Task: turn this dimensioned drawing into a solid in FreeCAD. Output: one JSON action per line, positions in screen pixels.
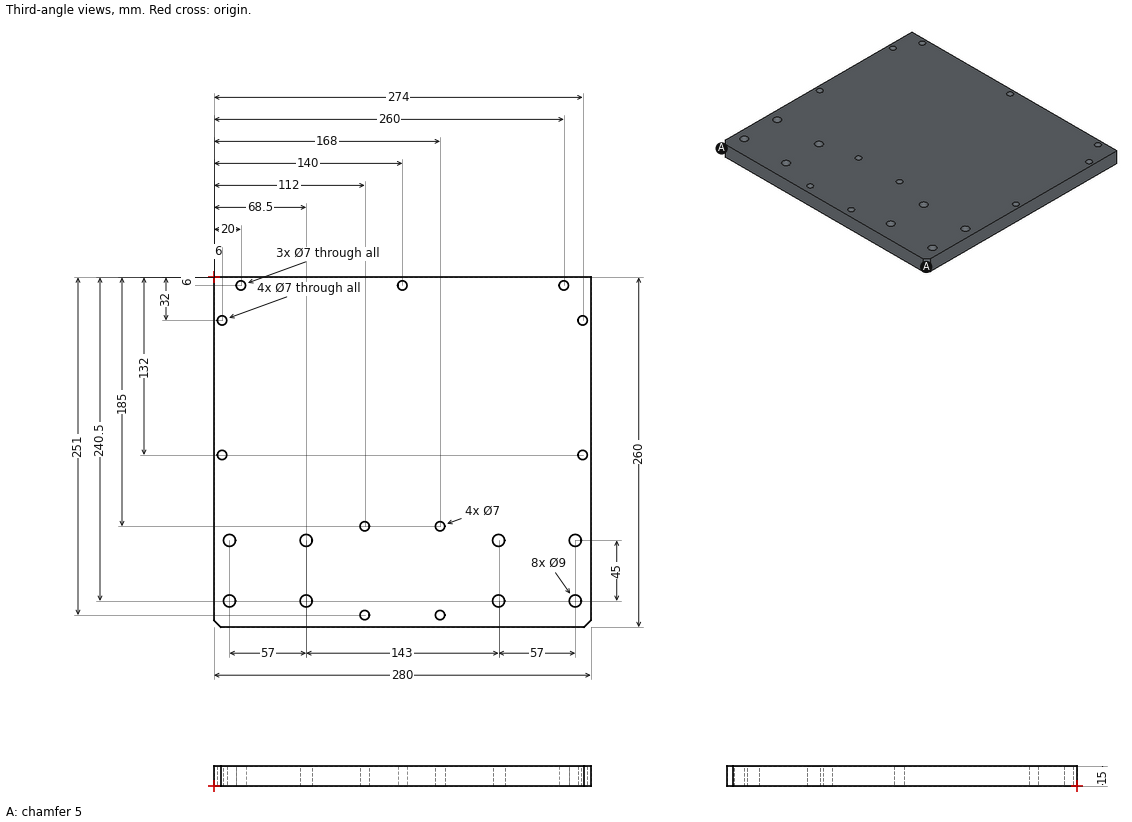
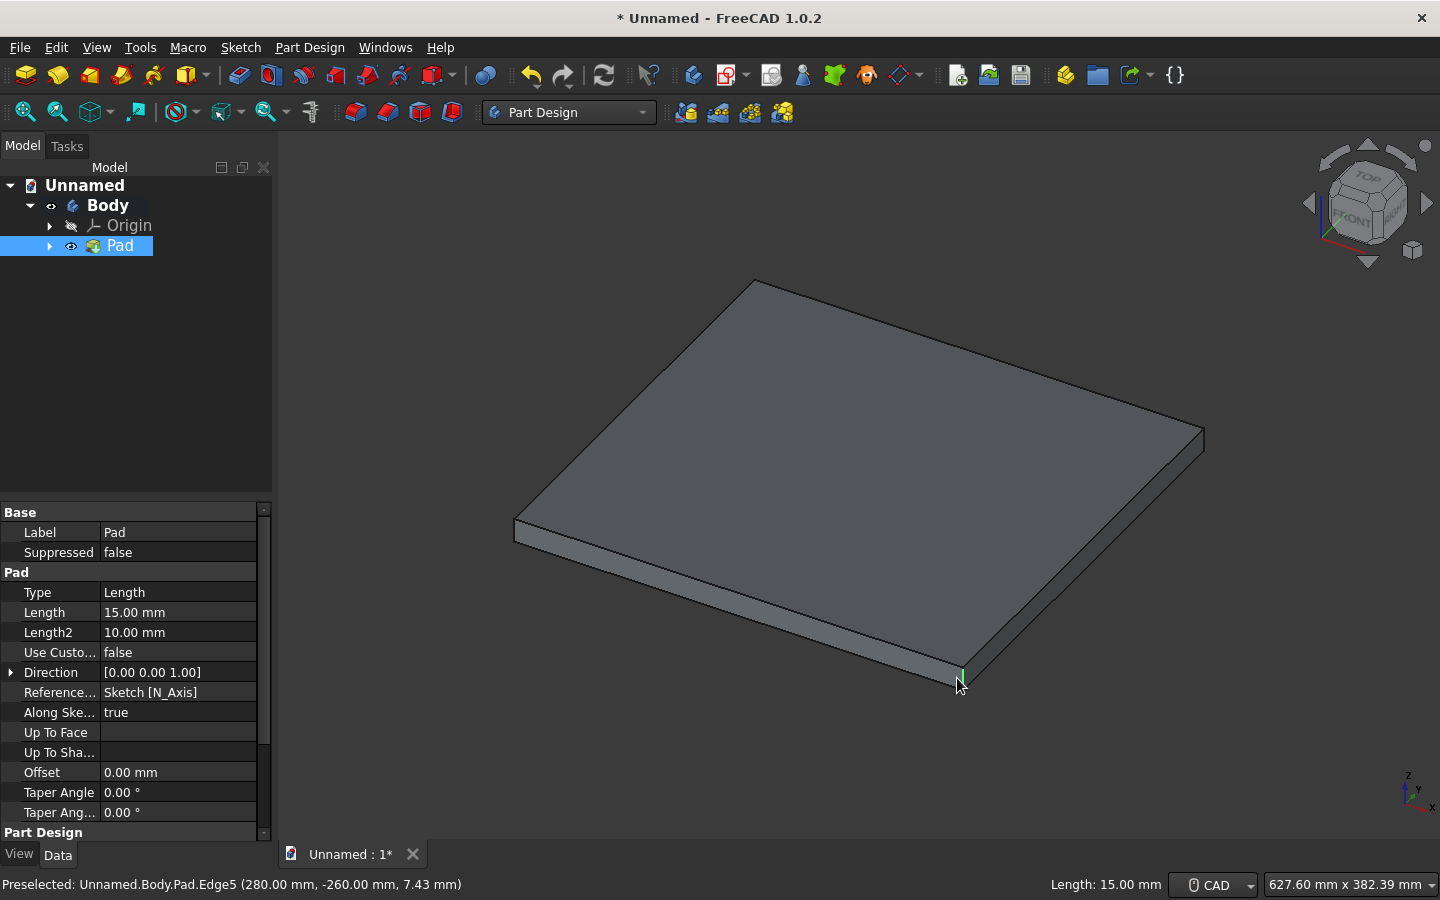
{"action": "key", "text": "0"}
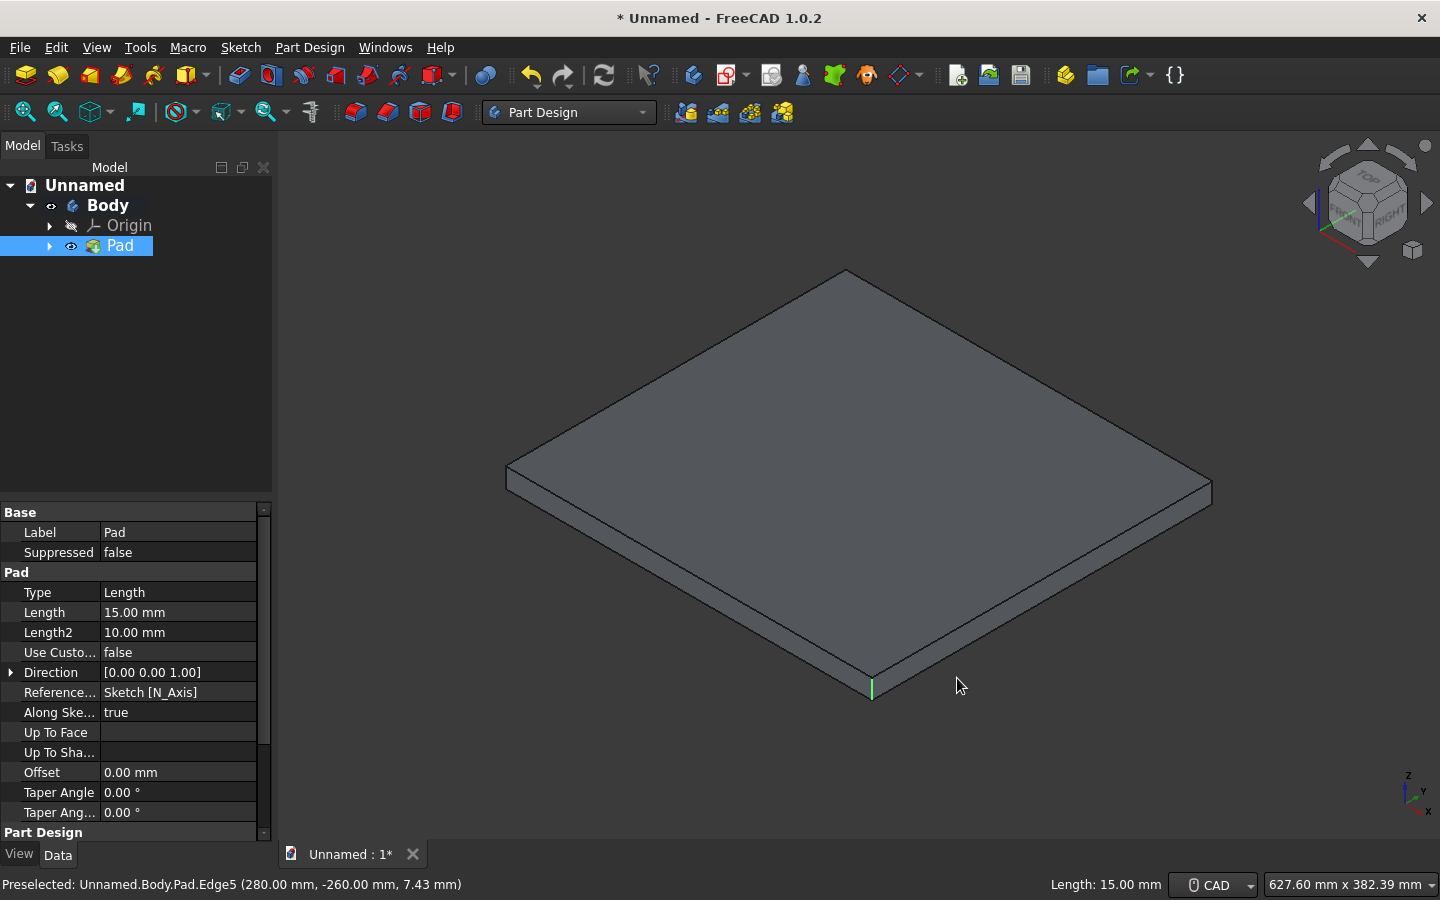
{"action": "key", "text": "2"}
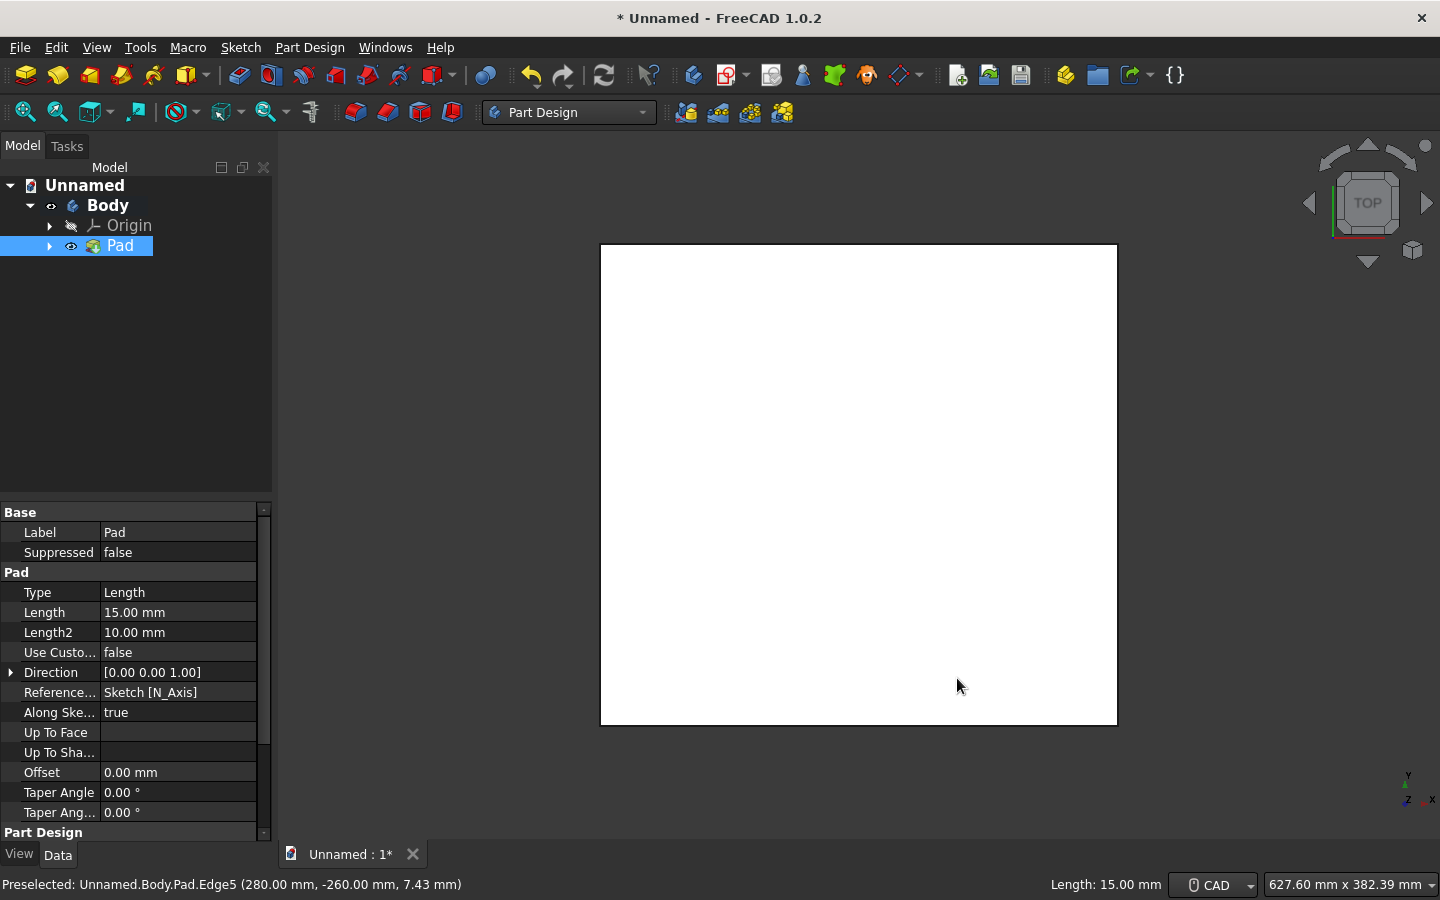
{"action": "key", "text": "1"}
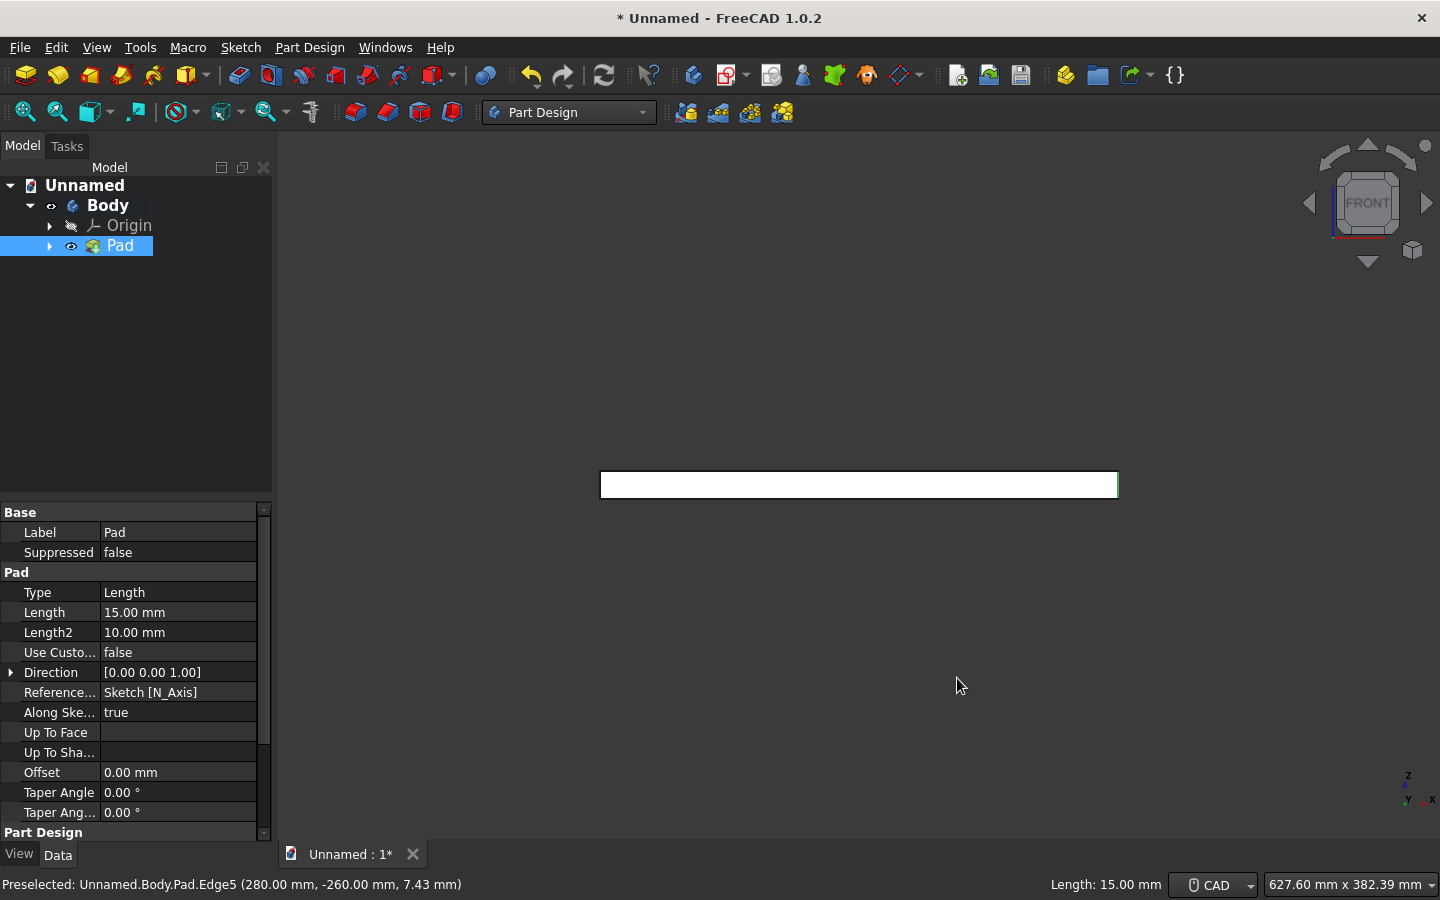
{"action": "left_click", "coordinate": [26, 112]}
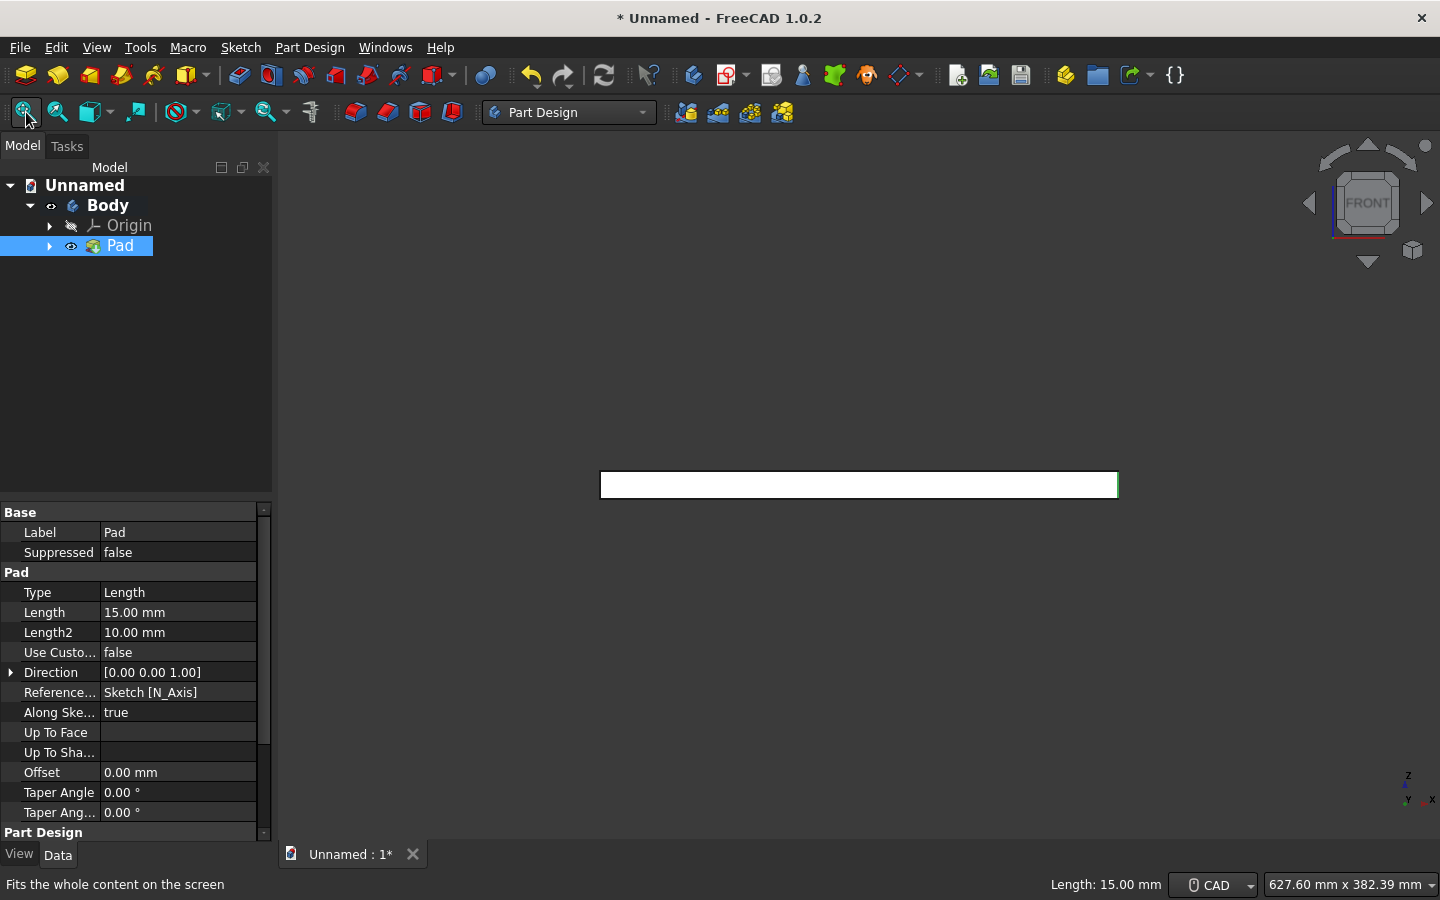
{"action": "left_click", "coordinate": [600, 484], "text": "ctrl"}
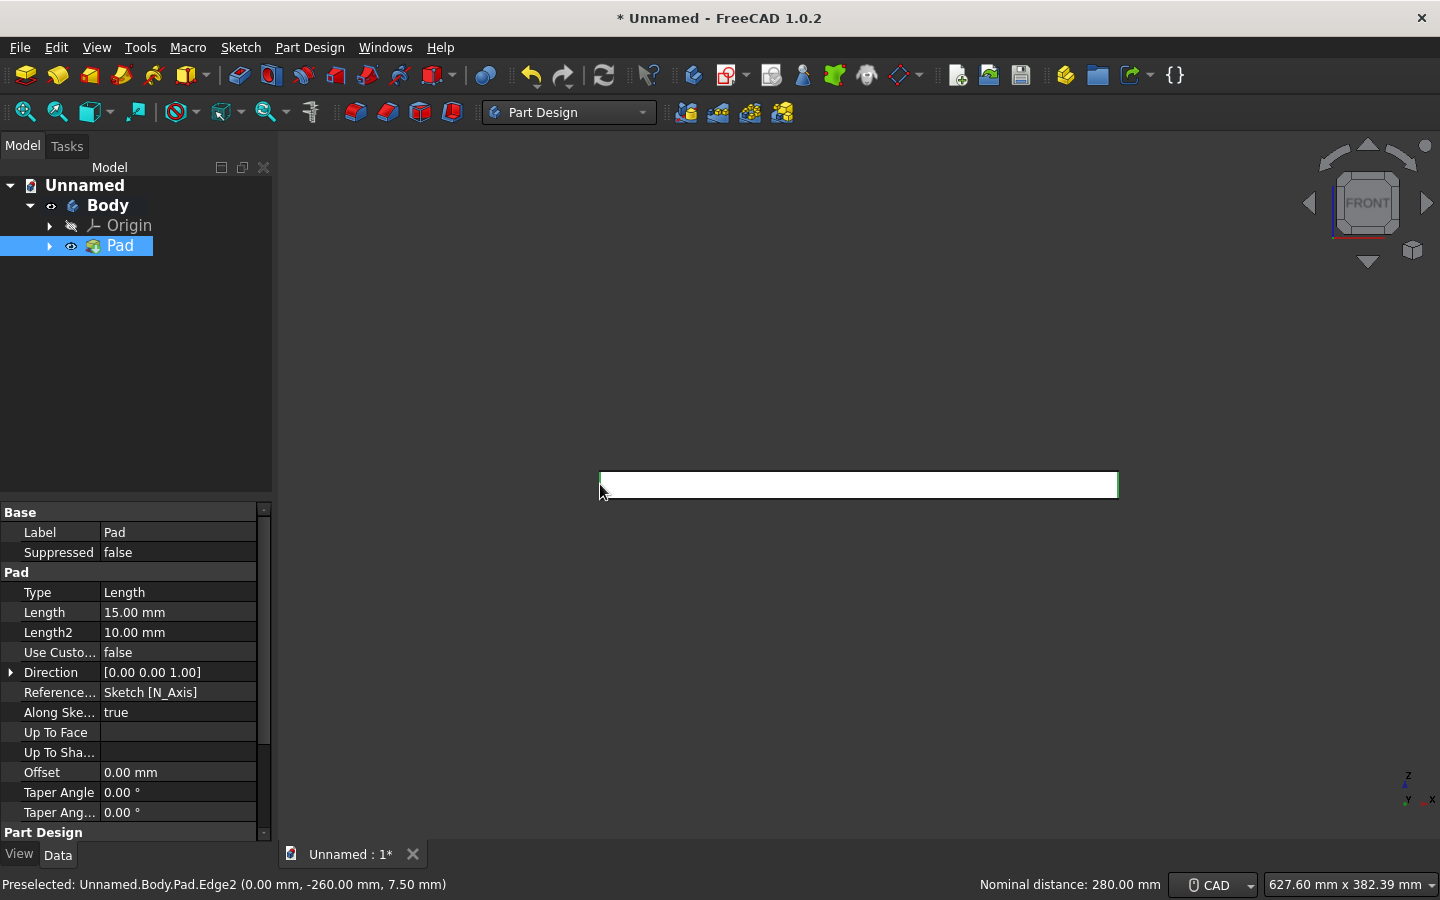
{"action": "left_click", "coordinate": [388, 112]}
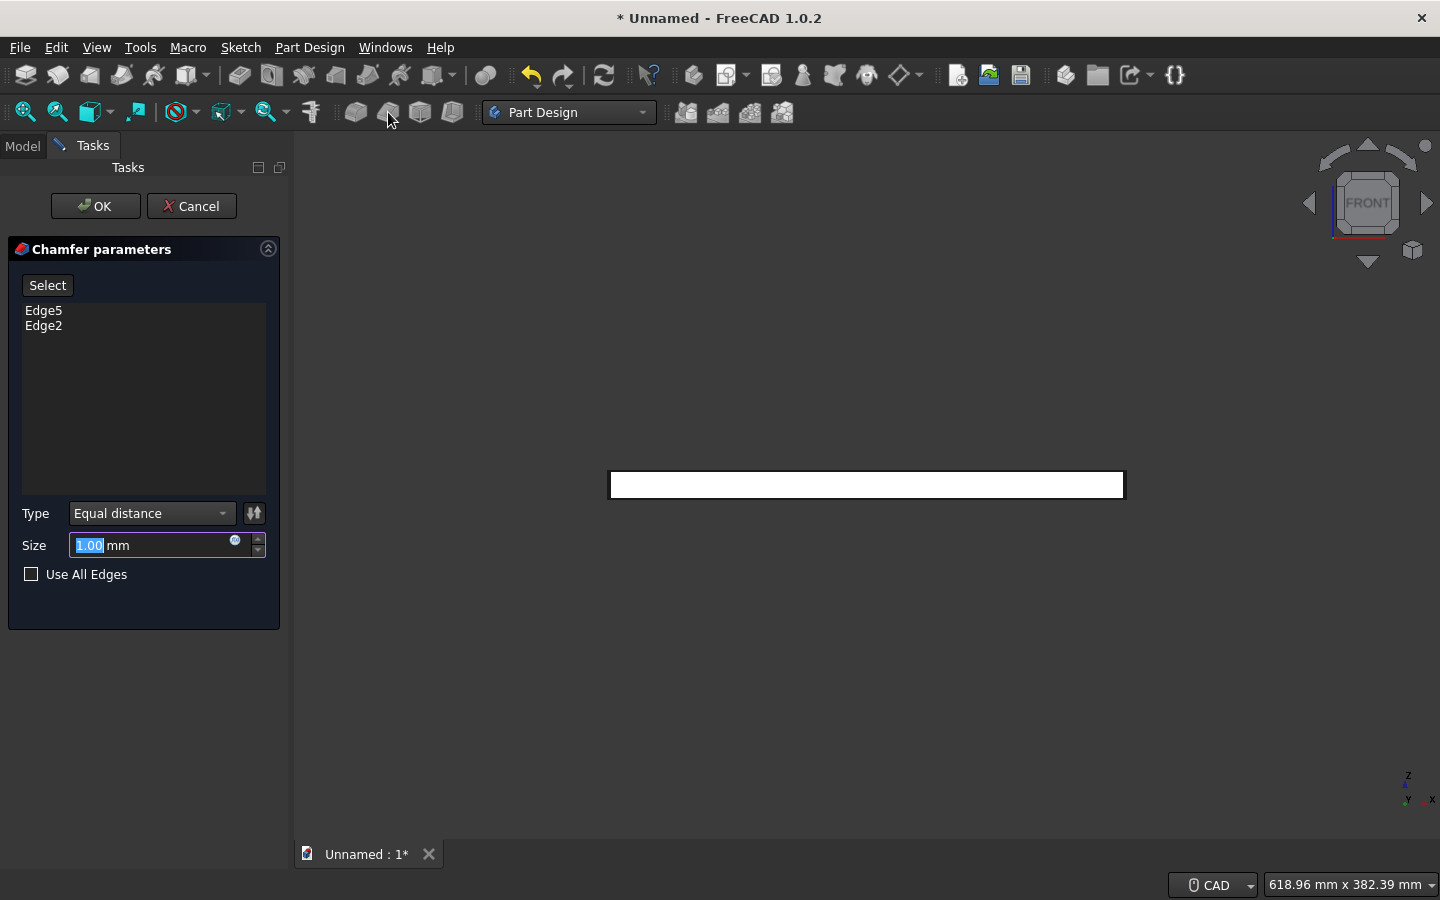
{"action": "type", "text": "5"}
{"action": "key", "text": "Tab"}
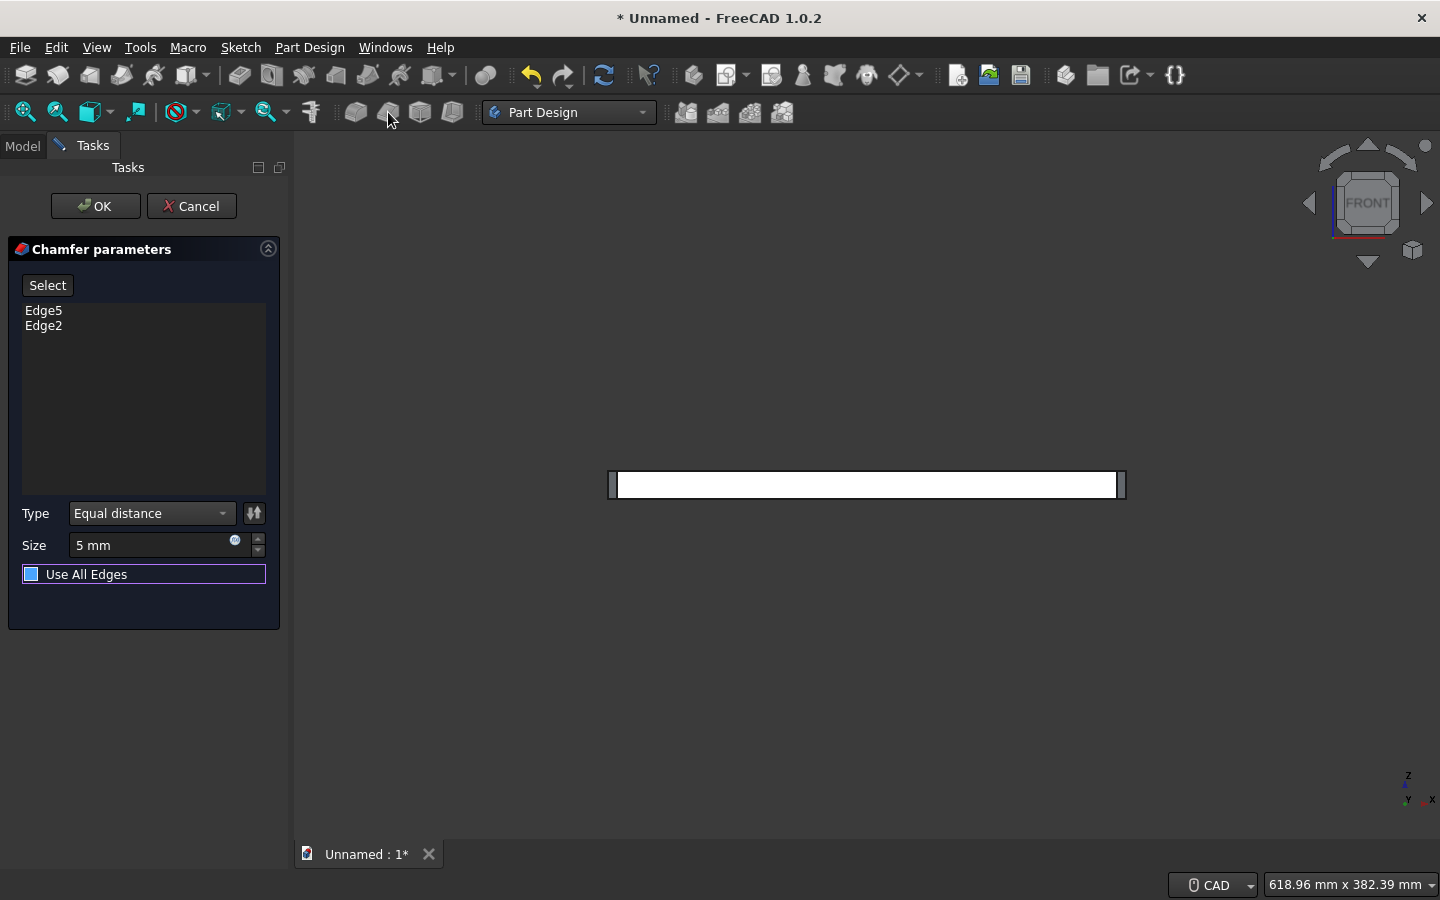
{"action": "left_click", "coordinate": [96, 206]}